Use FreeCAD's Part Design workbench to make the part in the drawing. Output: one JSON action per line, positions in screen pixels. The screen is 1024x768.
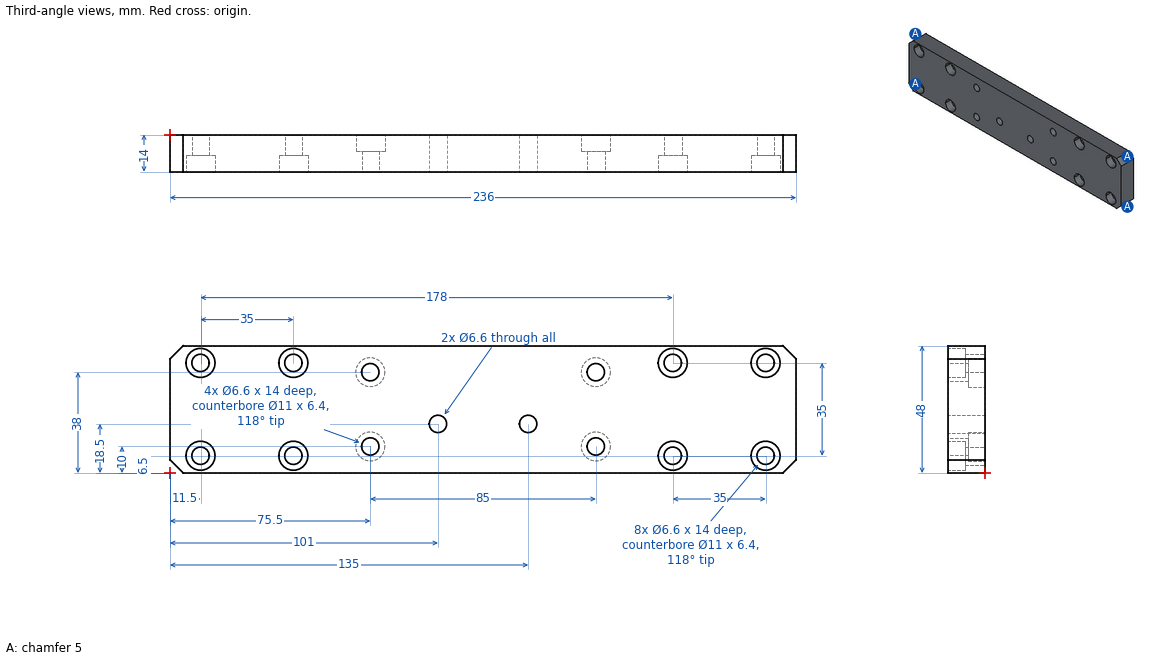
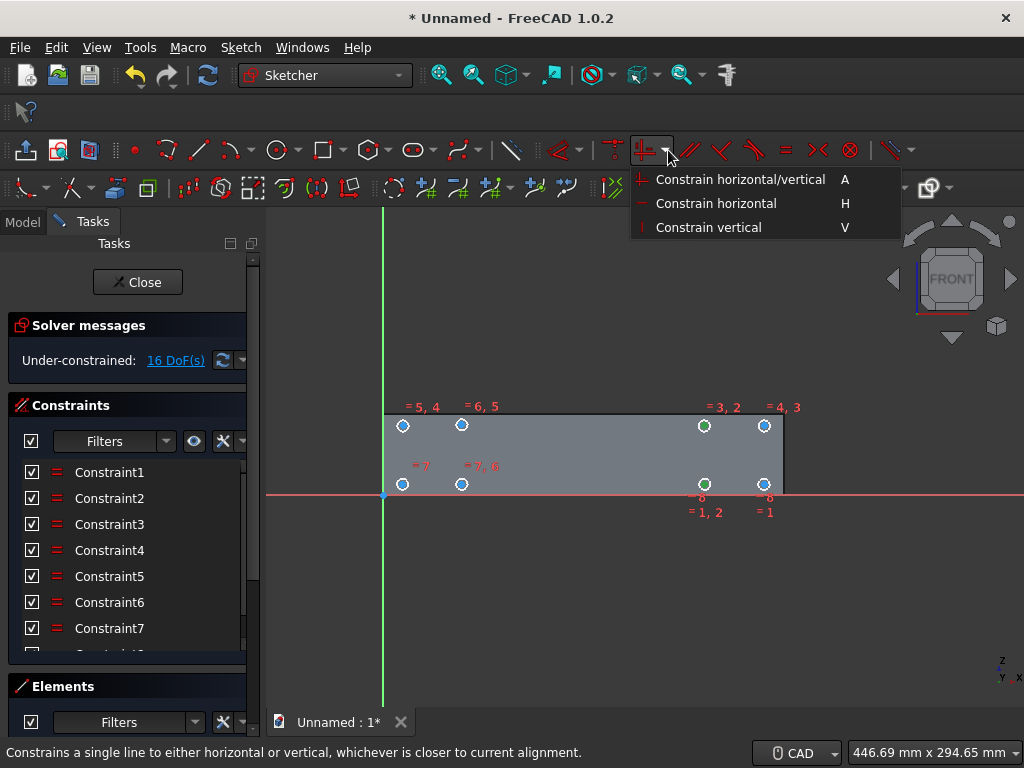
{"action": "left_click", "coordinate": [766, 227]}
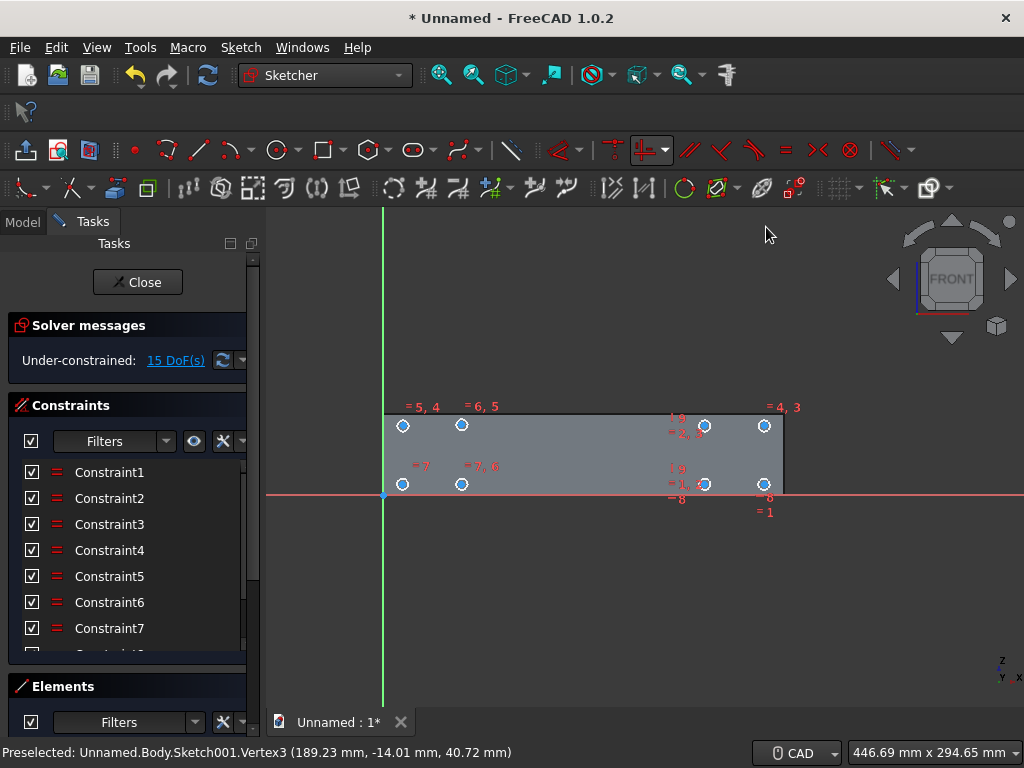
{"action": "left_click", "coordinate": [764, 484]}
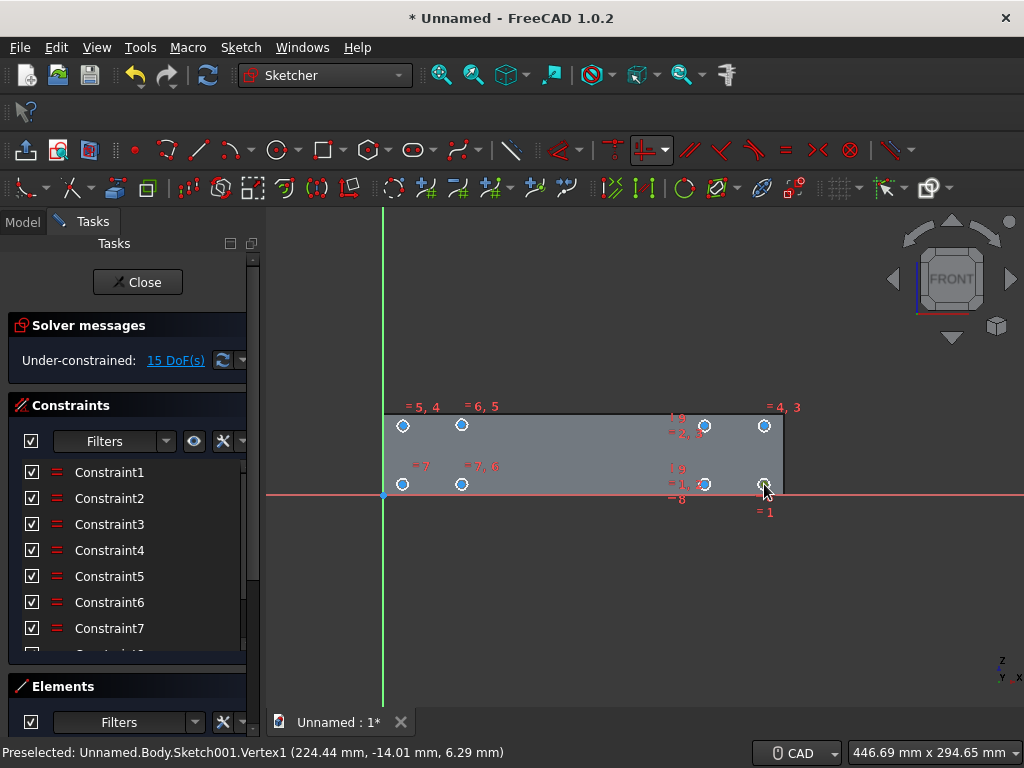
{"action": "left_click", "coordinate": [764, 426]}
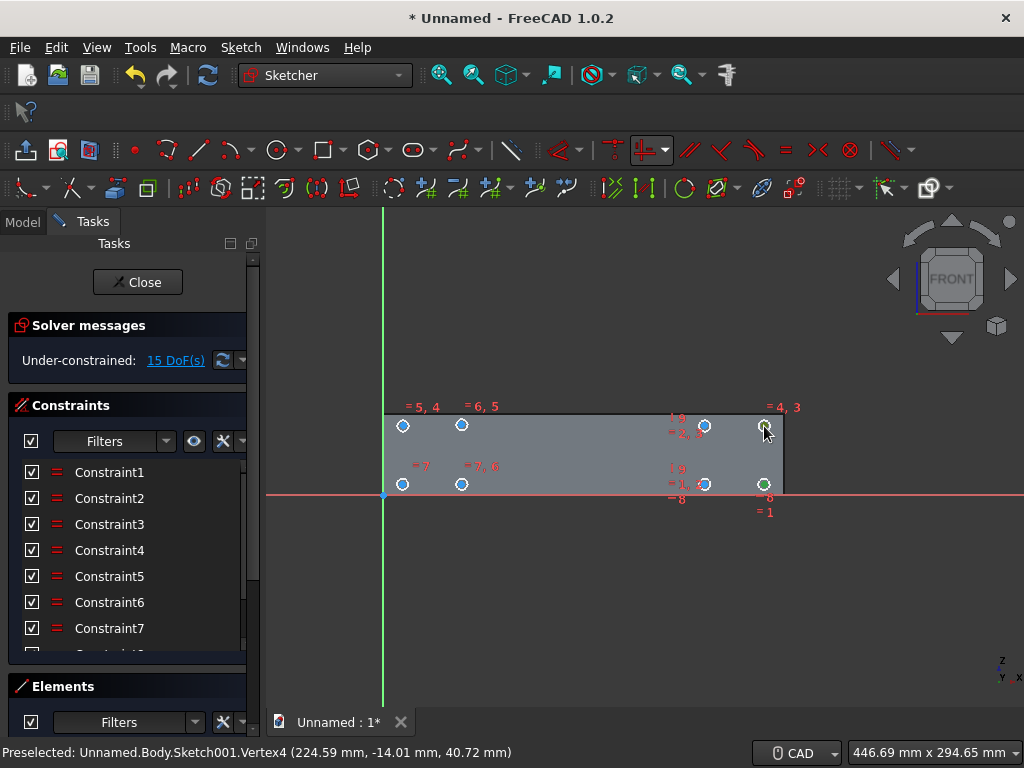
{"action": "left_click", "coordinate": [668, 150]}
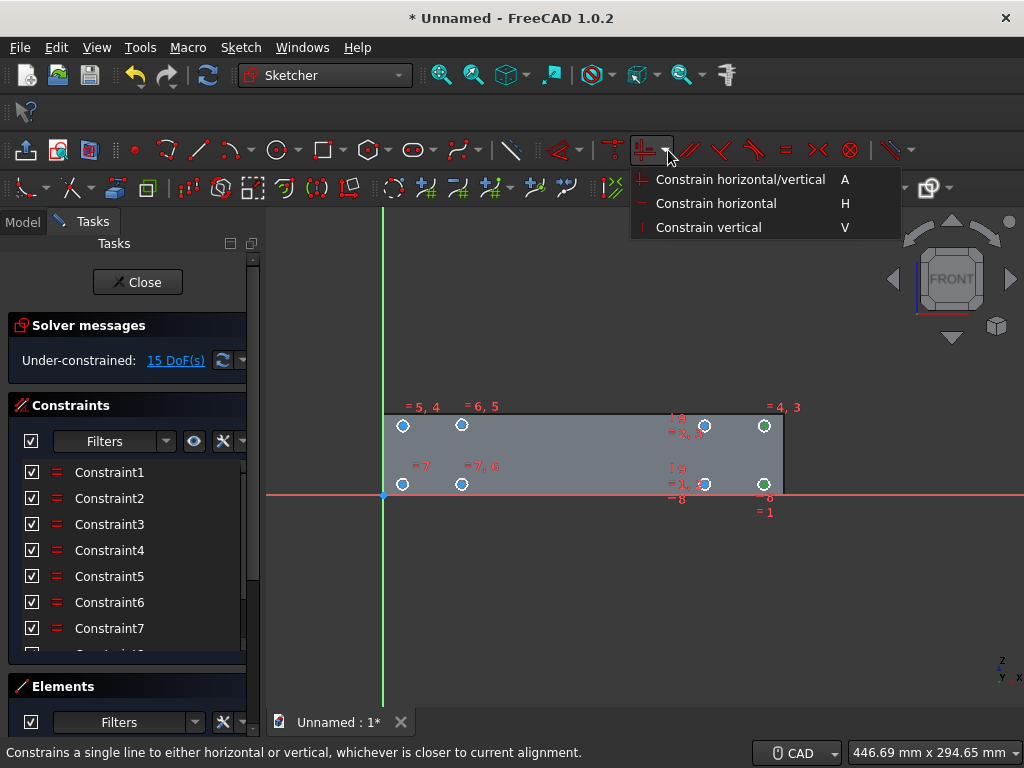
{"action": "left_click", "coordinate": [766, 227]}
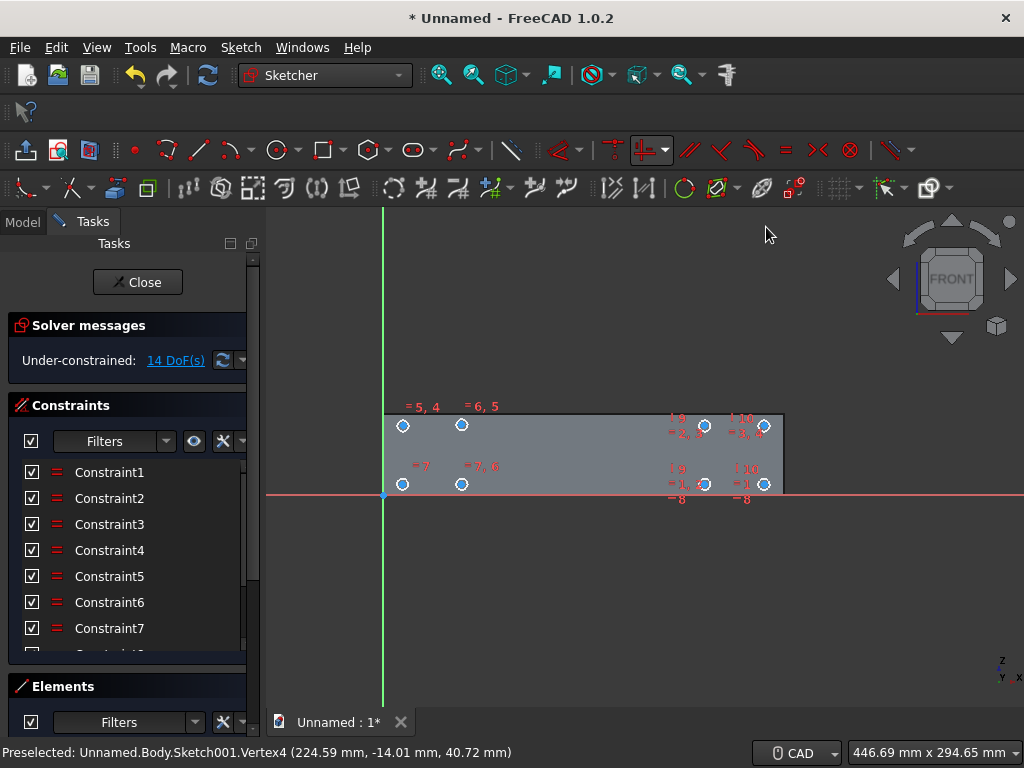
{"action": "left_click", "coordinate": [705, 426]}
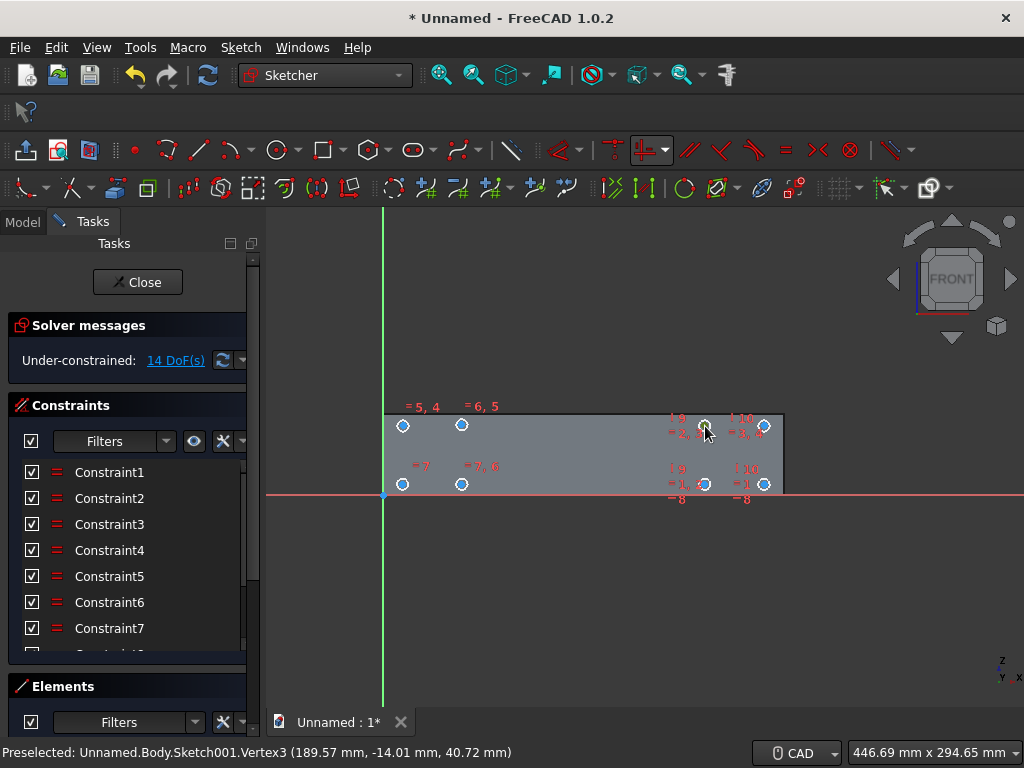
{"action": "left_click", "coordinate": [764, 426]}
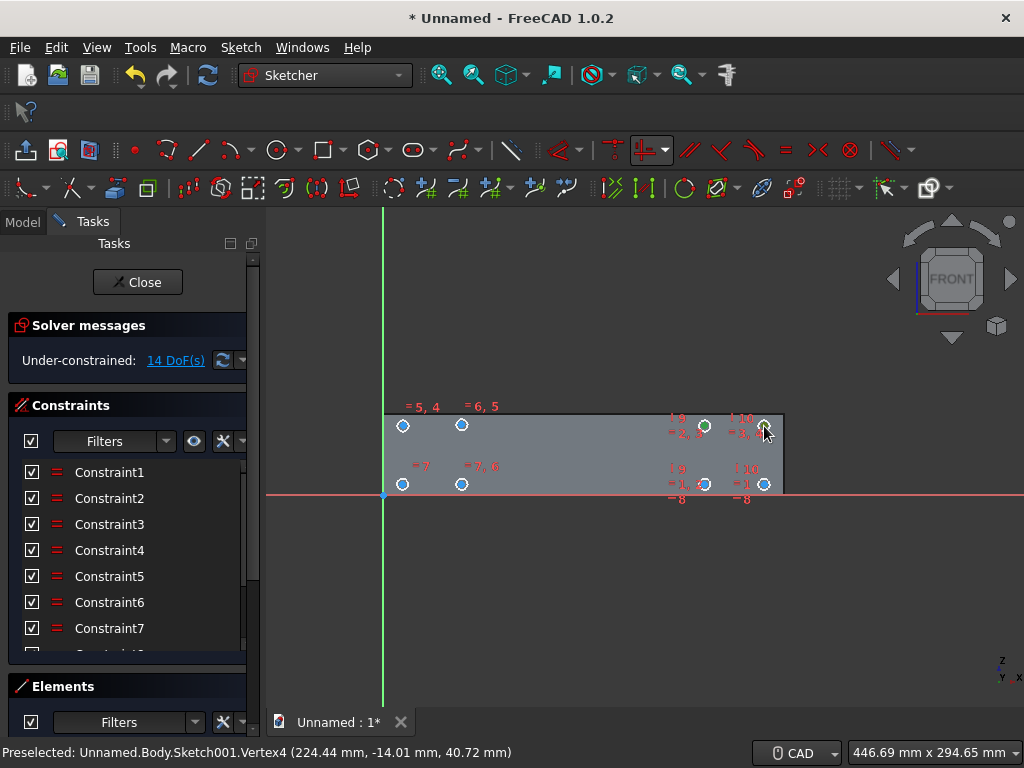
{"action": "key", "text": "h"}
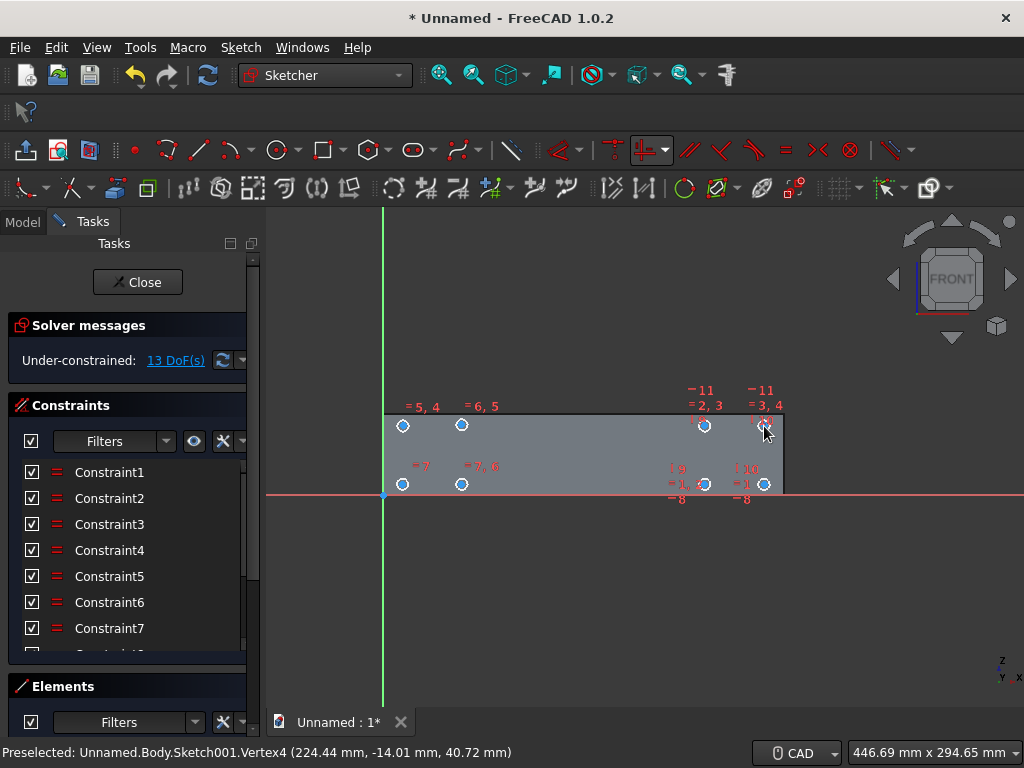
{"action": "left_click", "coordinate": [705, 426]}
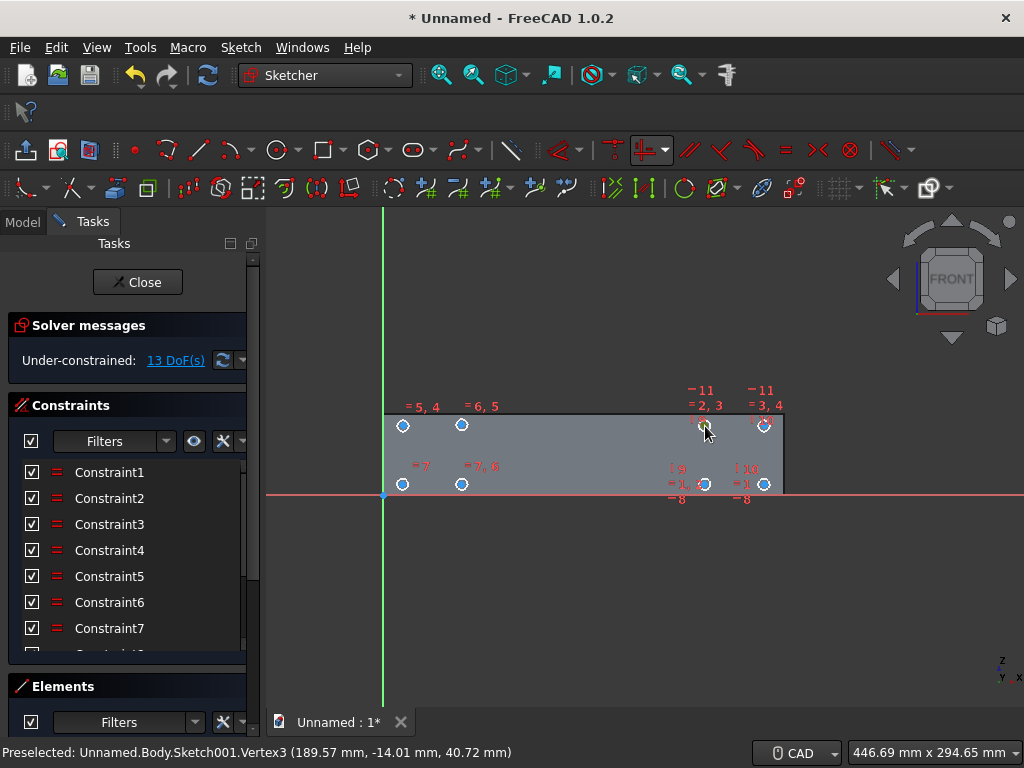
{"action": "left_click", "coordinate": [403, 426]}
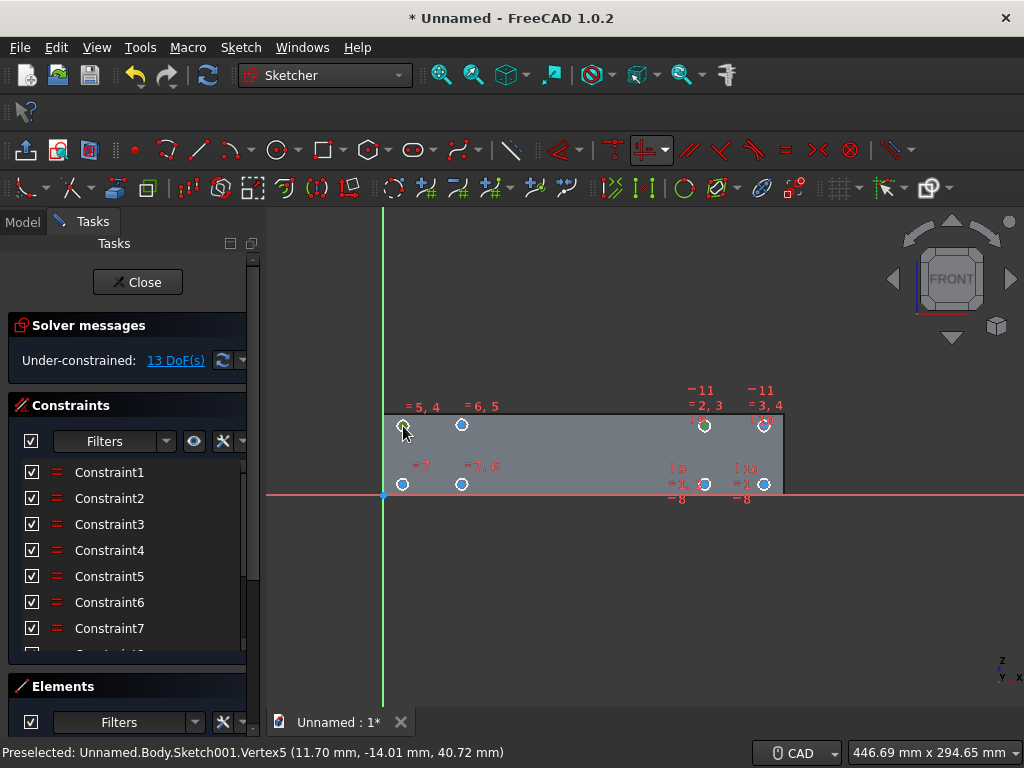
{"action": "left_click", "coordinate": [668, 150]}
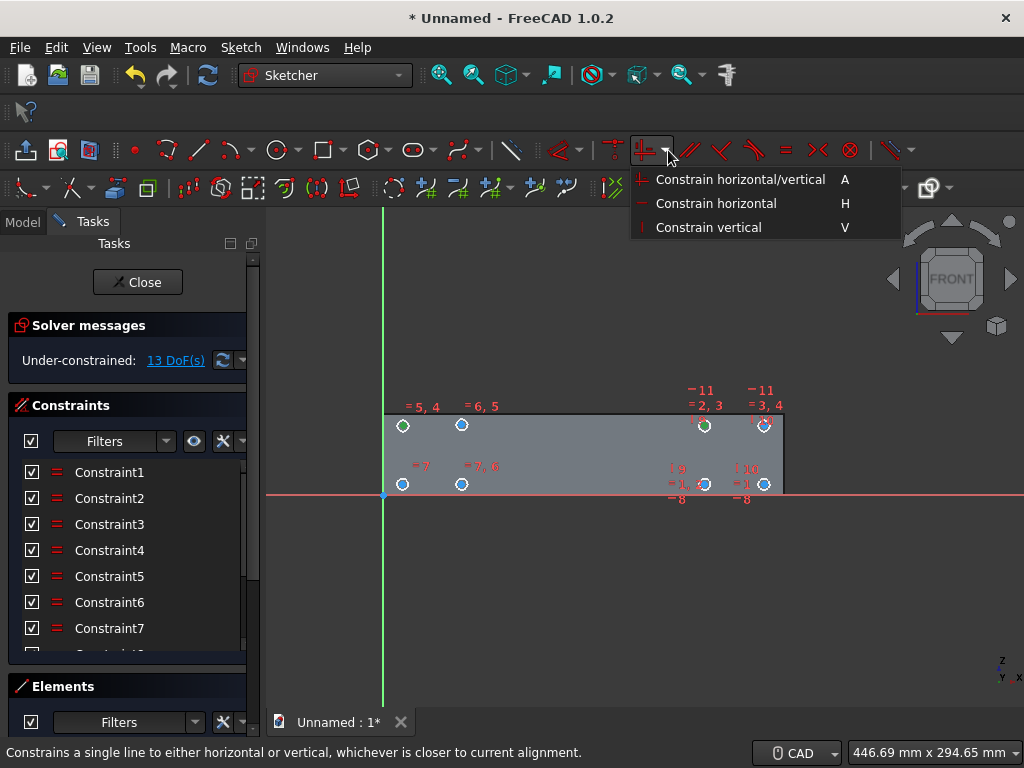
{"action": "left_click", "coordinate": [766, 203]}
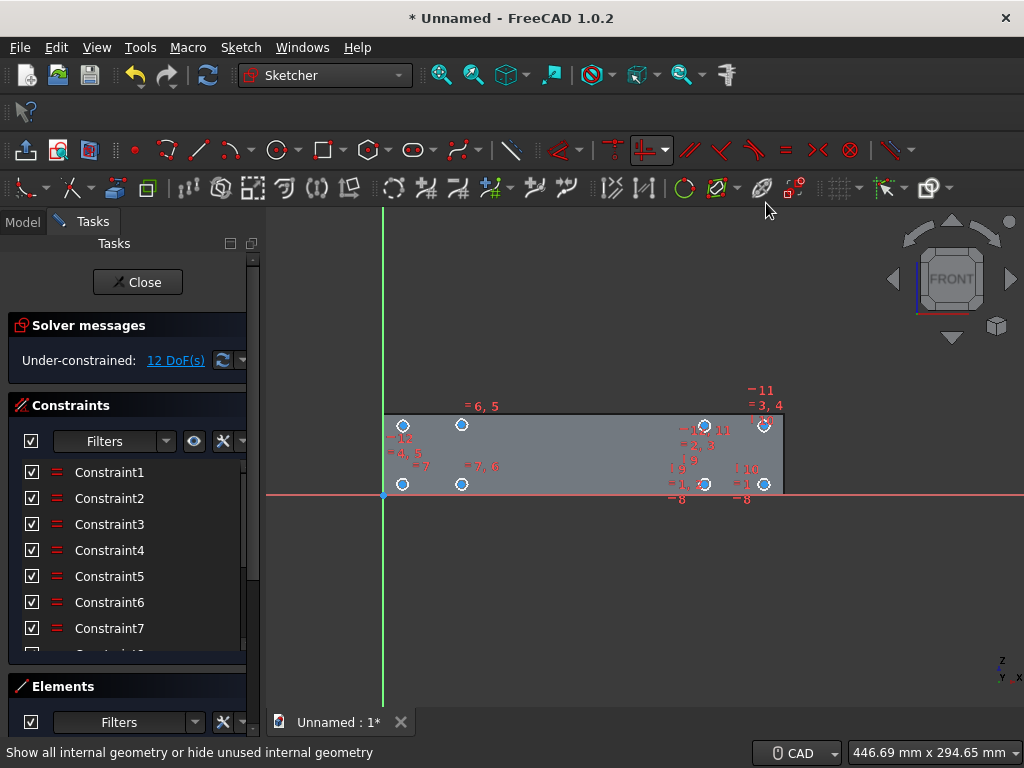
{"action": "left_click", "coordinate": [403, 426]}